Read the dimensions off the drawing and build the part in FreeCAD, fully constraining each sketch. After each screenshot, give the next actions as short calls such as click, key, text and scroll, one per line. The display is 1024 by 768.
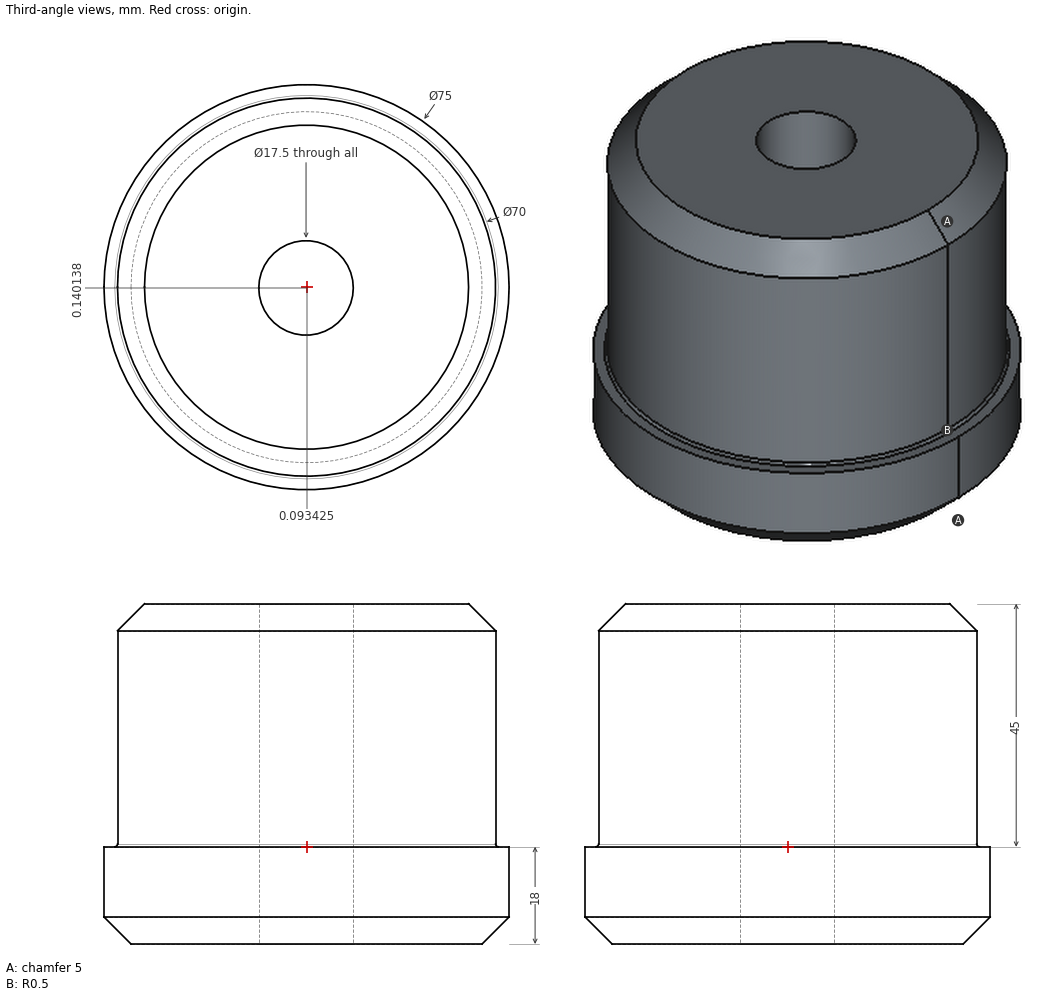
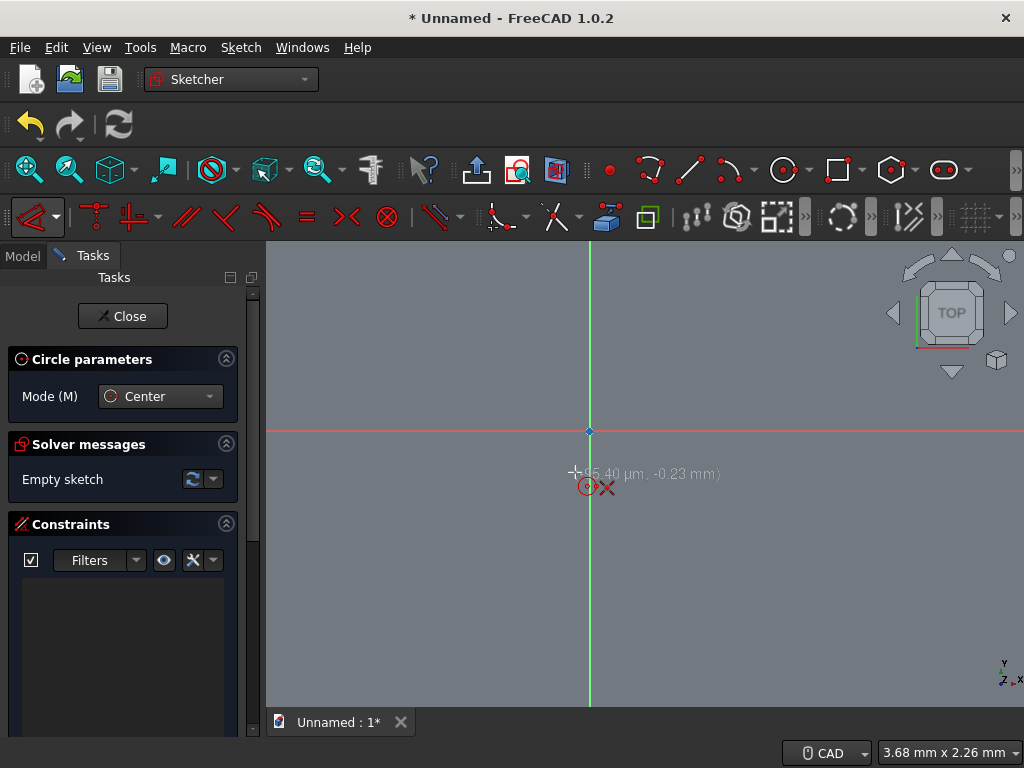
click(570, 460)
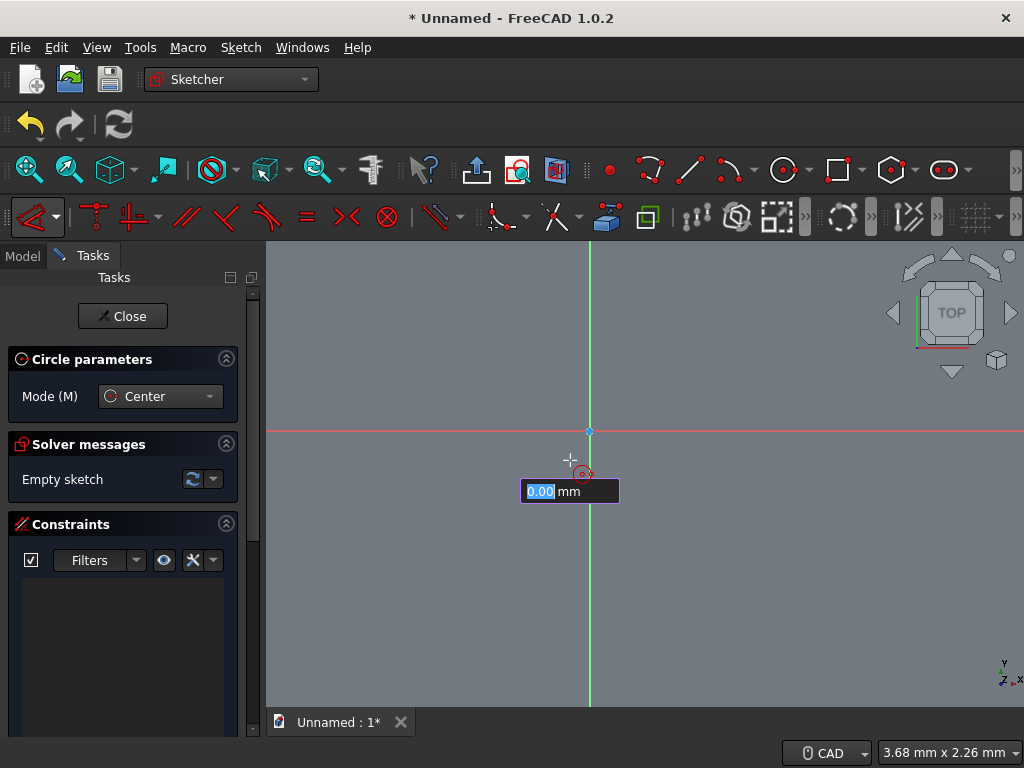
scroll(577, 475, down, 13)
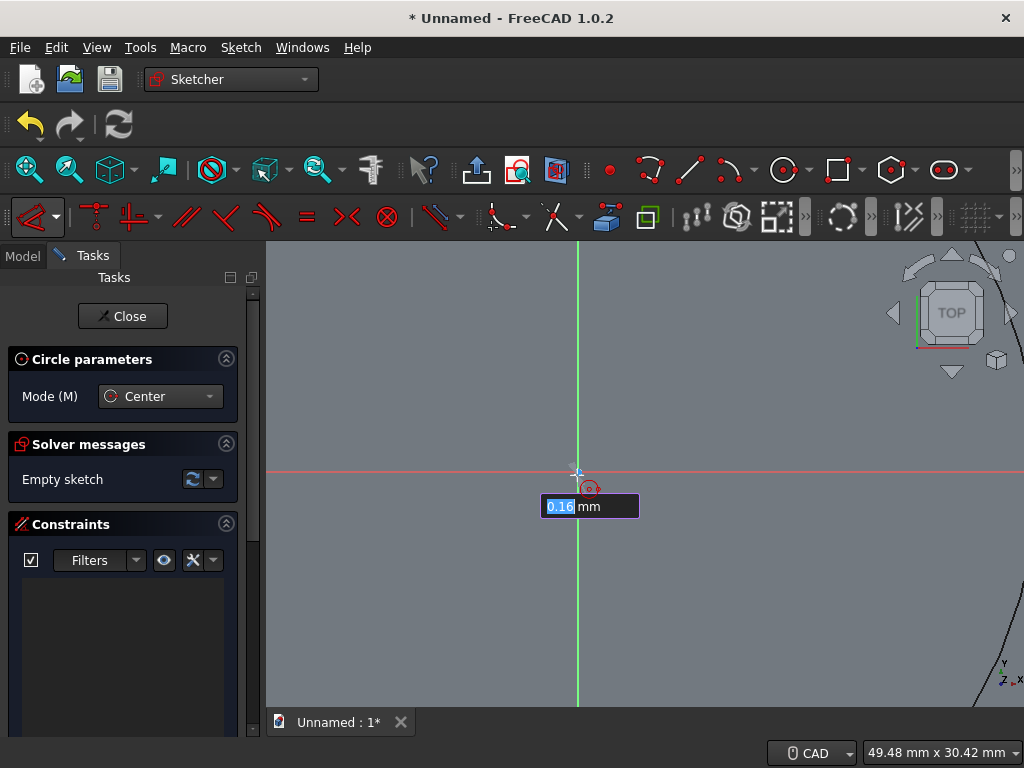
click(672, 380)
key(Escape)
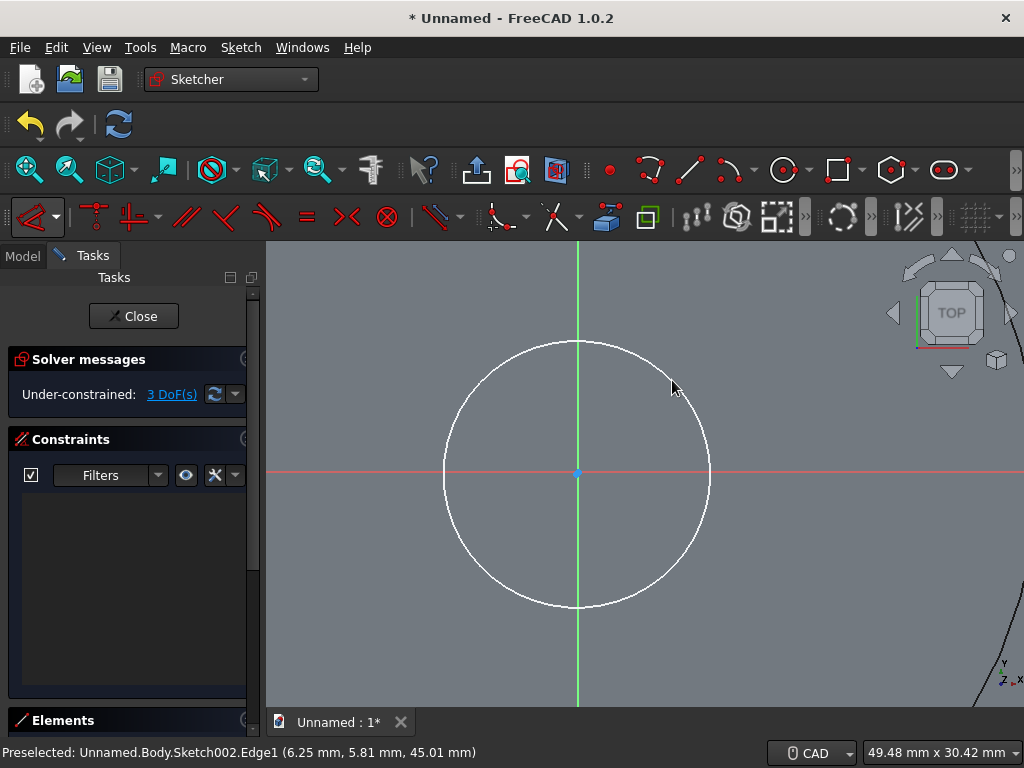
click(671, 380)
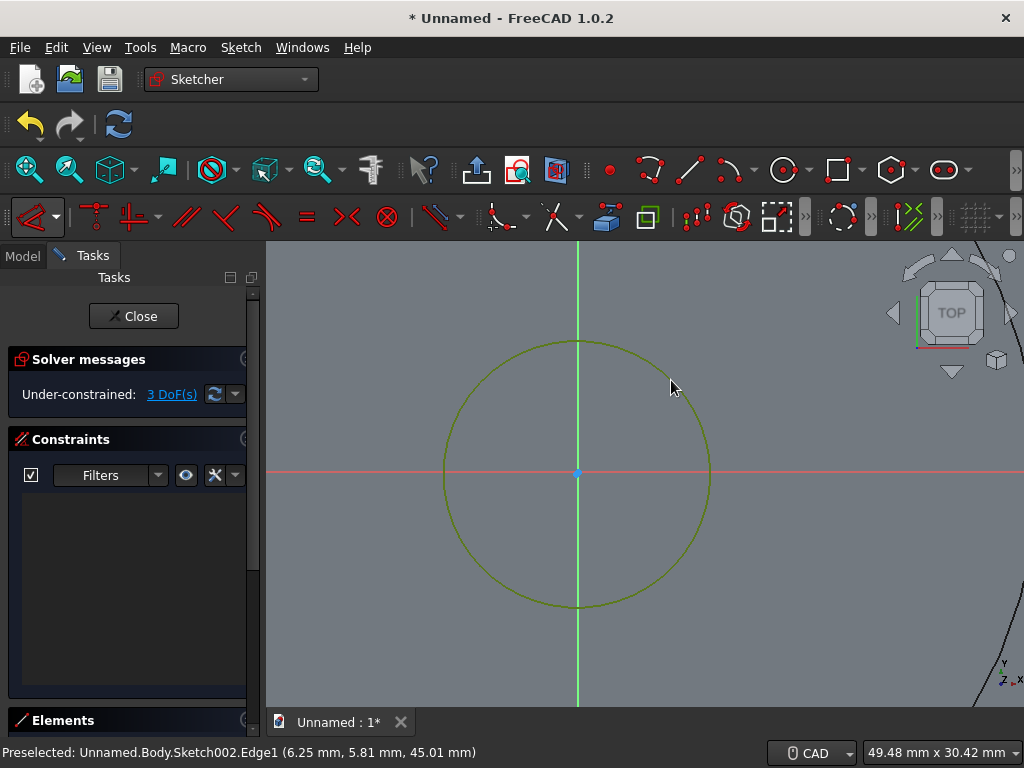
click(58, 218)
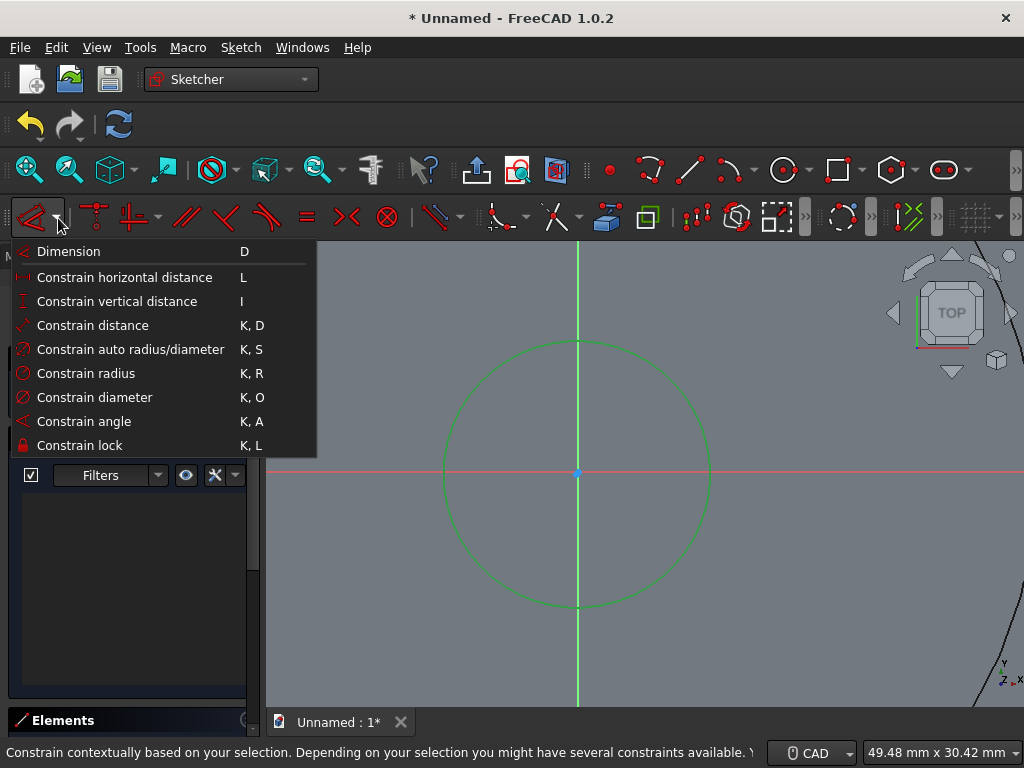
click(164, 397)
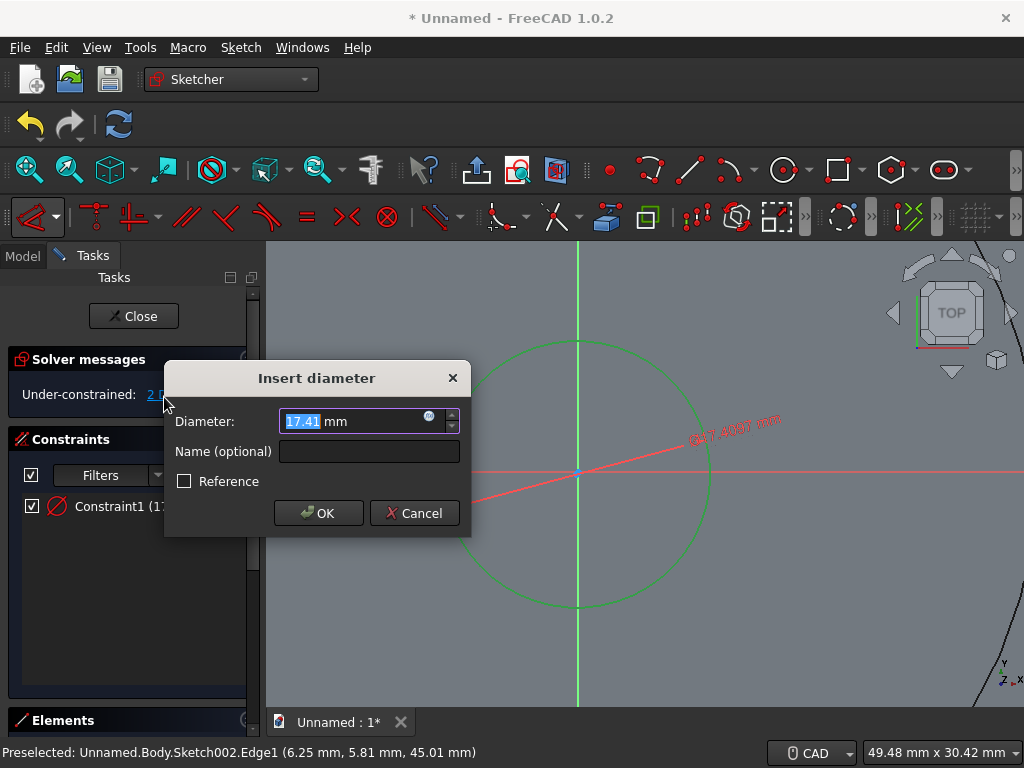
text(17.5)
key(Return)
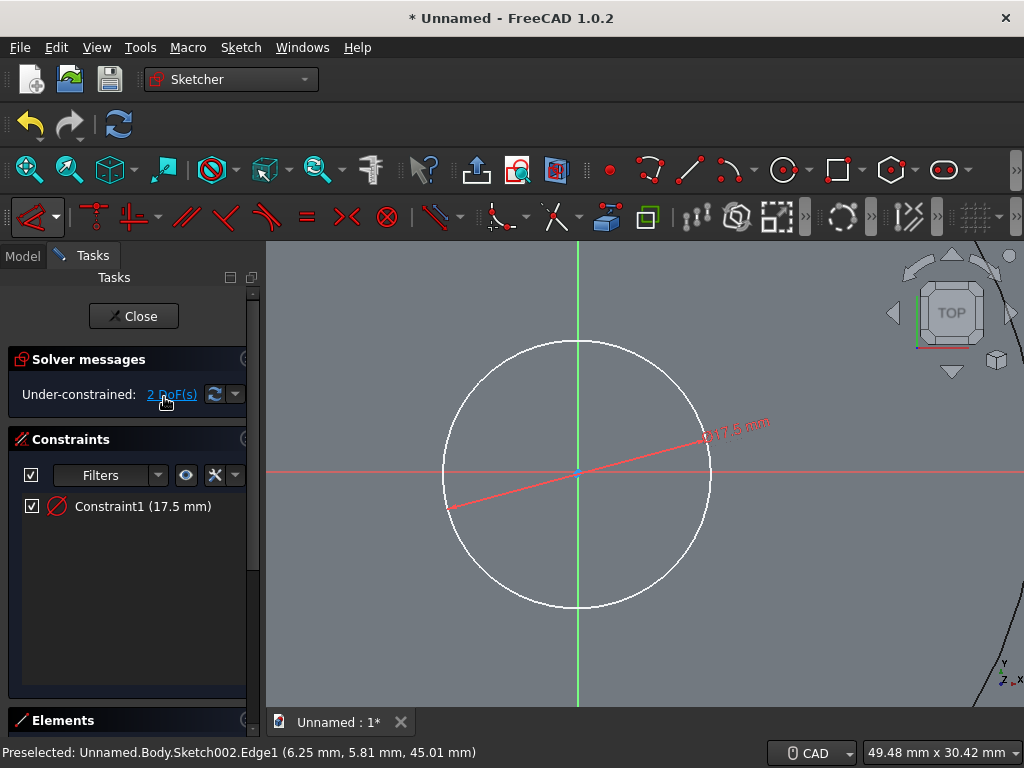
scroll(577, 474, up, 17)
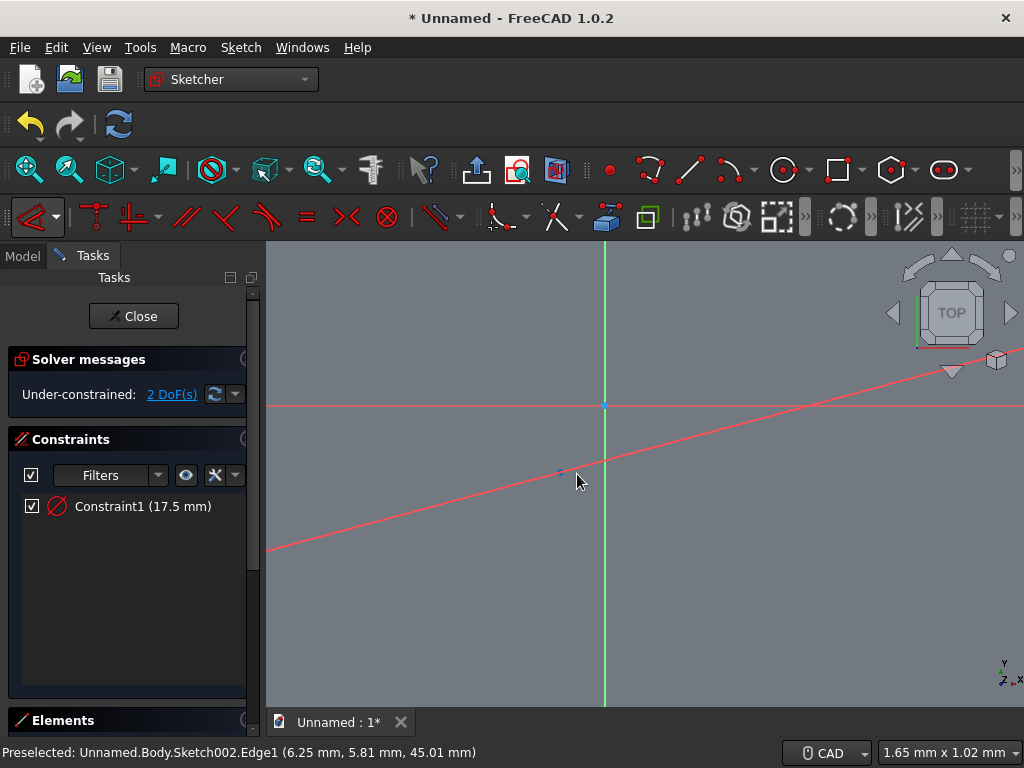
click(561, 472)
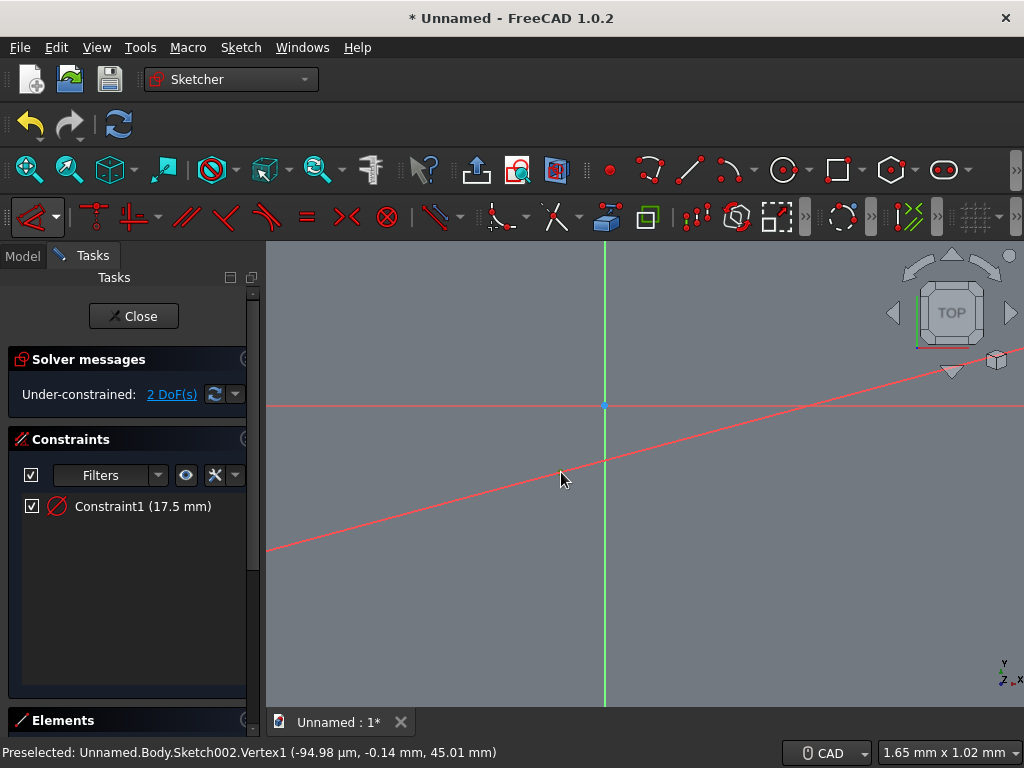
click(58, 218)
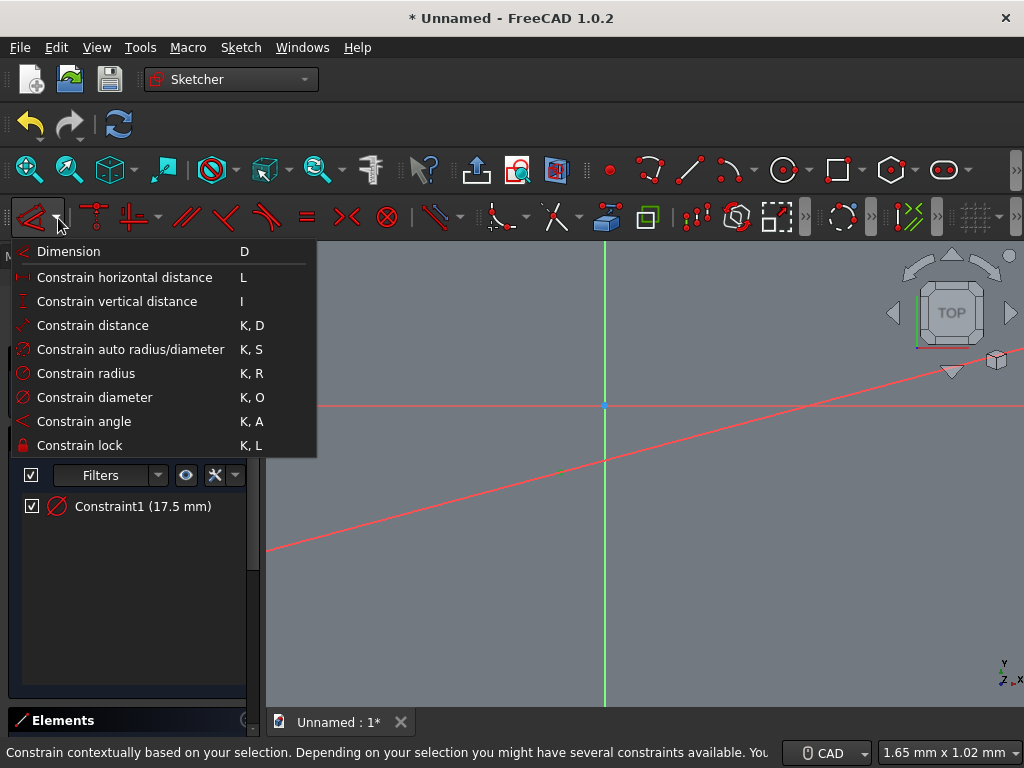
click(164, 277)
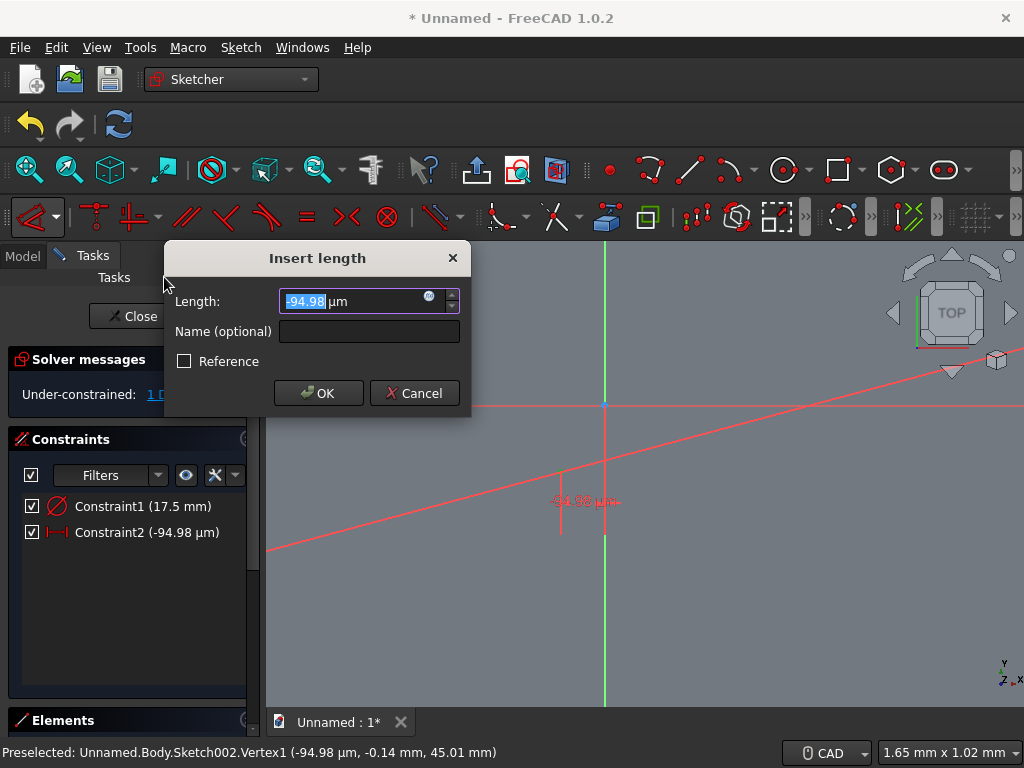
key(ctrl+a)
text(-0.093425 mm)
key(Return)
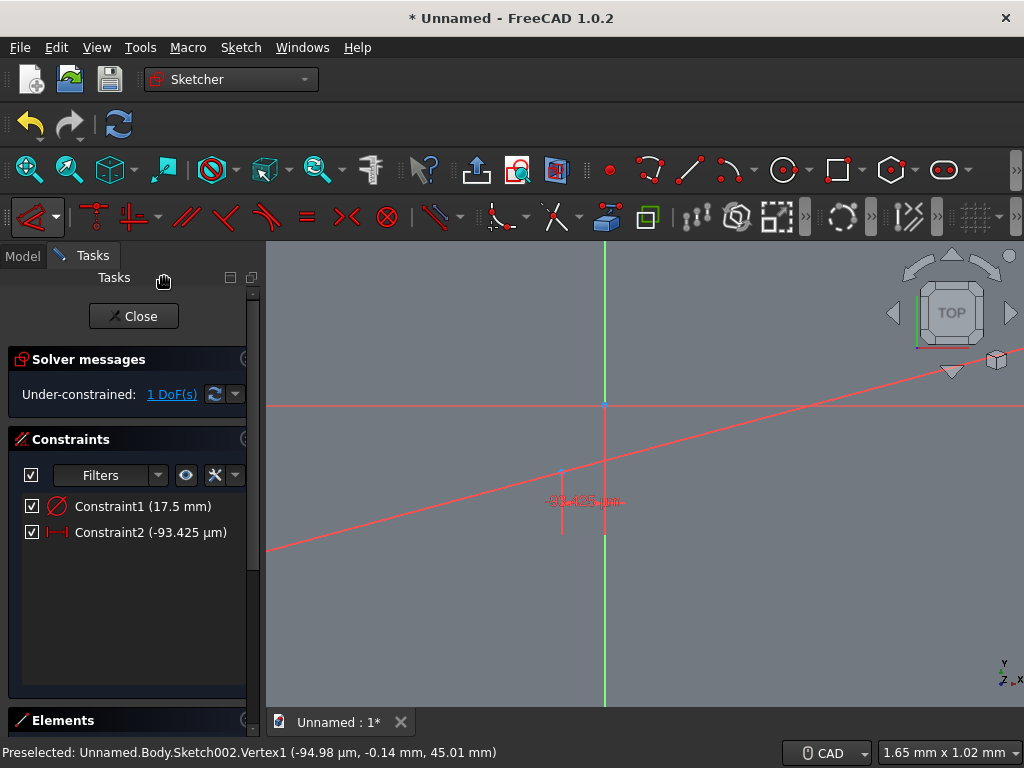
click(562, 472)